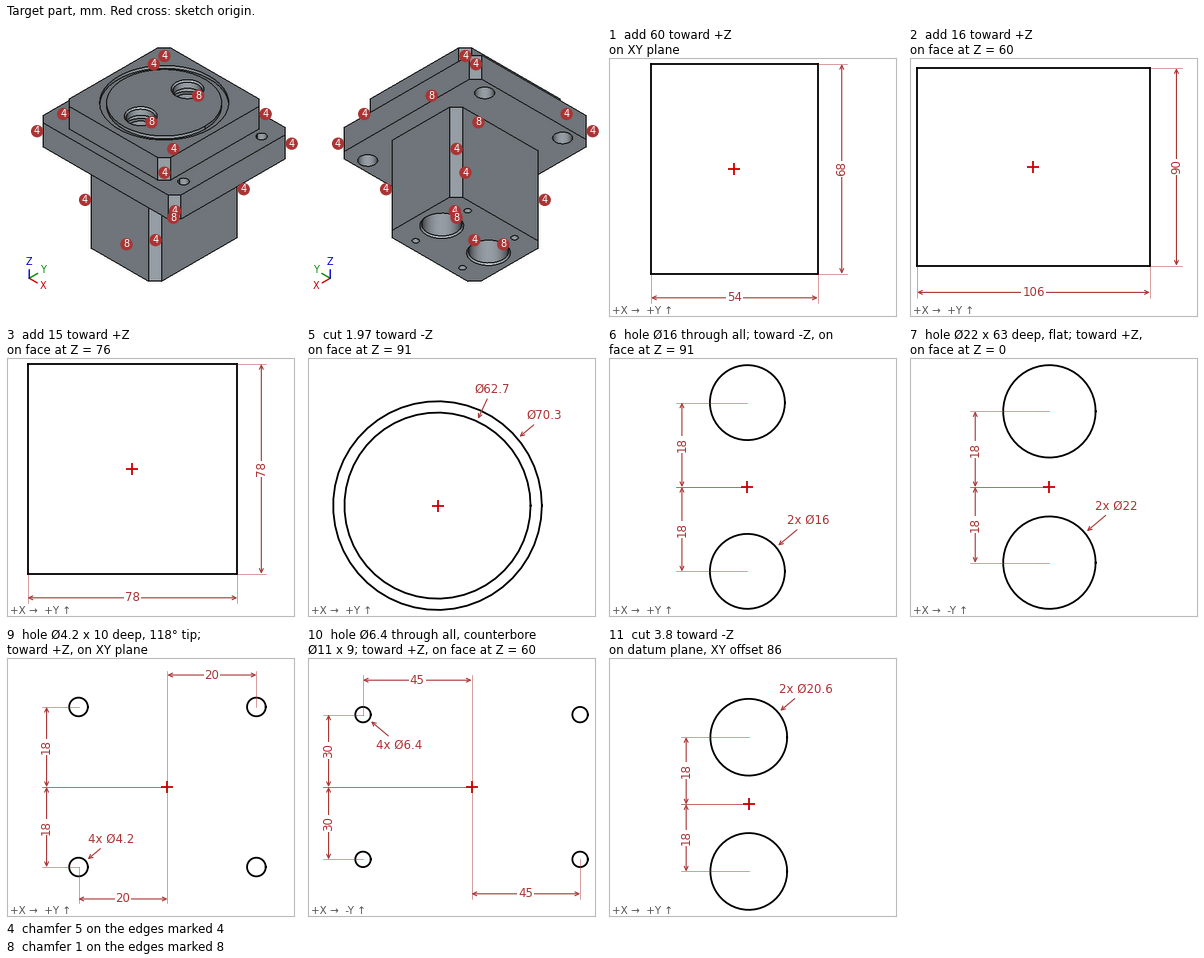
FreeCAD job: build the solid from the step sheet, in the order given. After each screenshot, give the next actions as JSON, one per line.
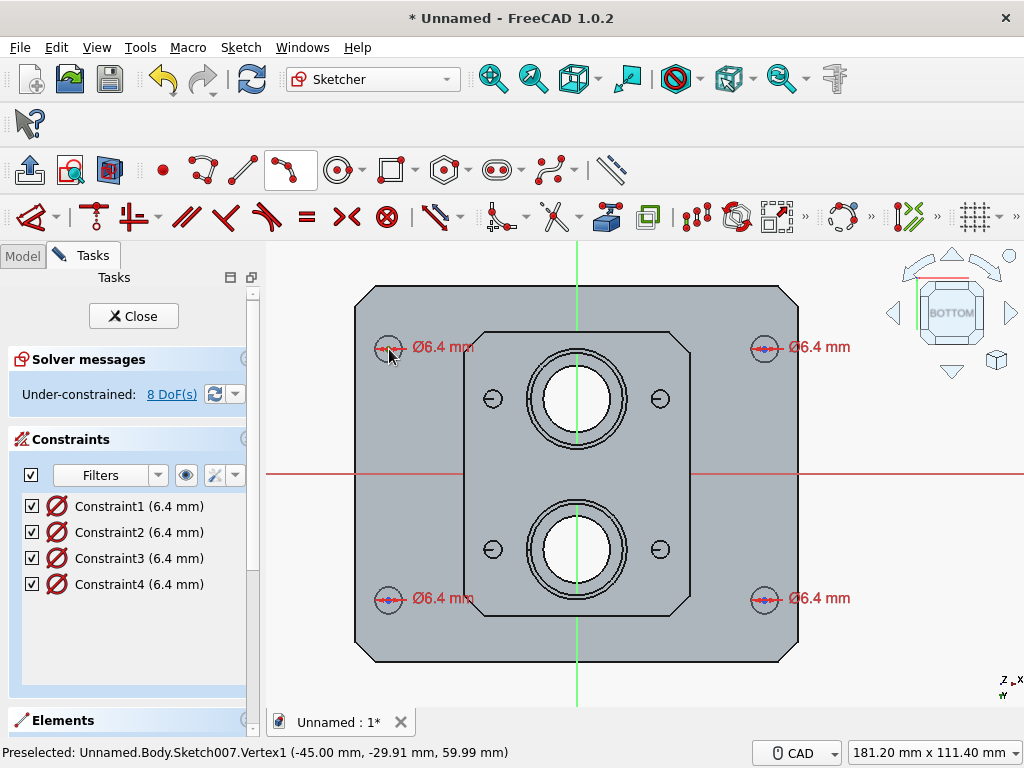
{"action": "left_click", "coordinate": [389, 600]}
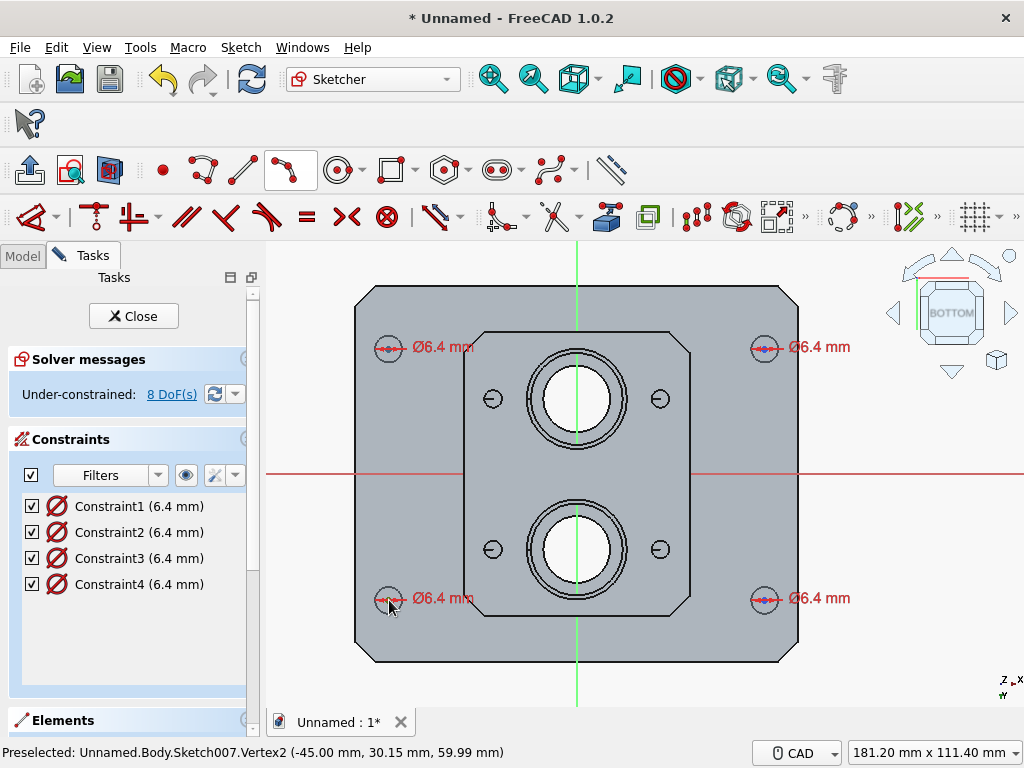
{"action": "key", "text": "v"}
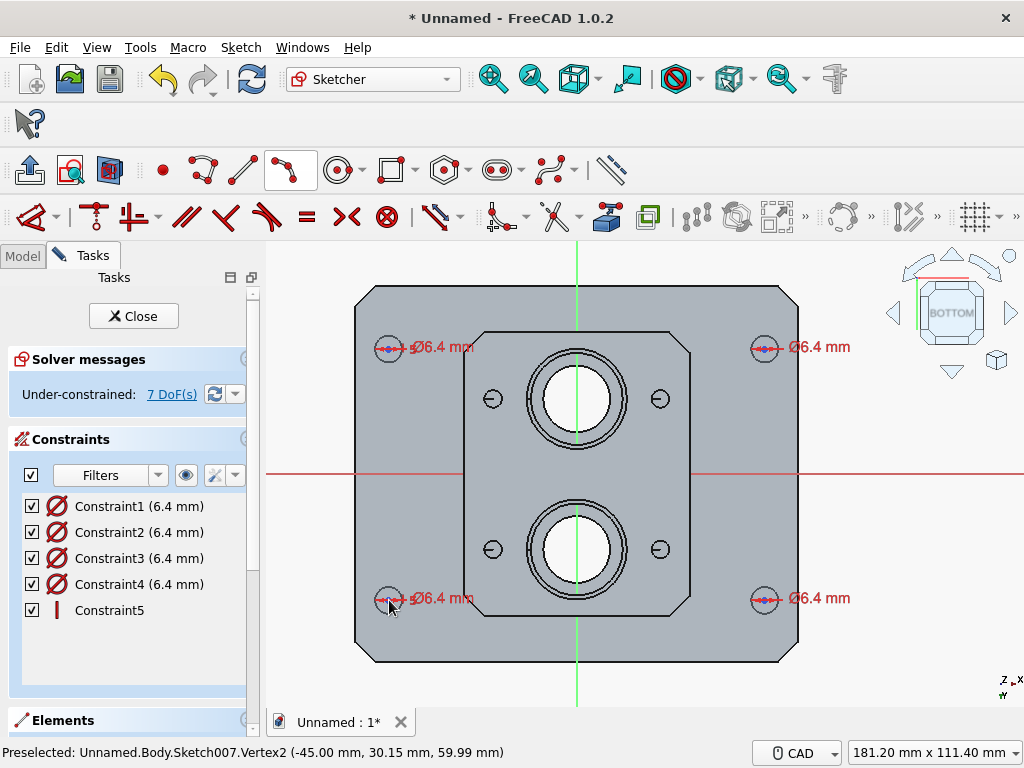
{"action": "left_click", "coordinate": [389, 600]}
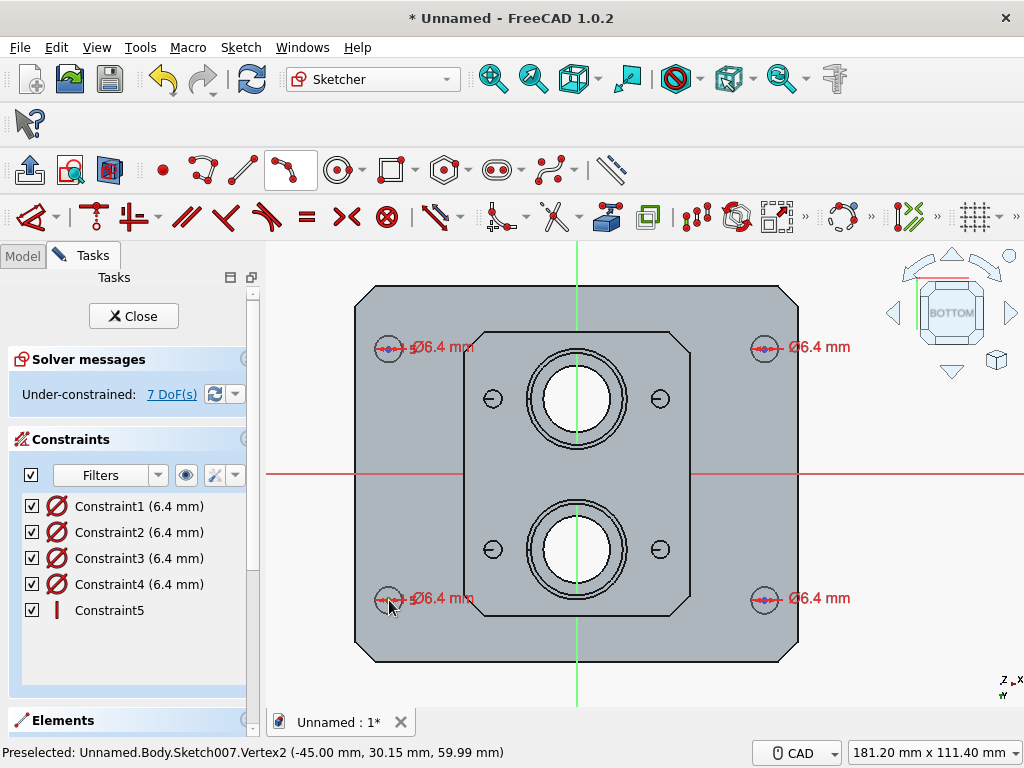
{"action": "left_click", "coordinate": [765, 600]}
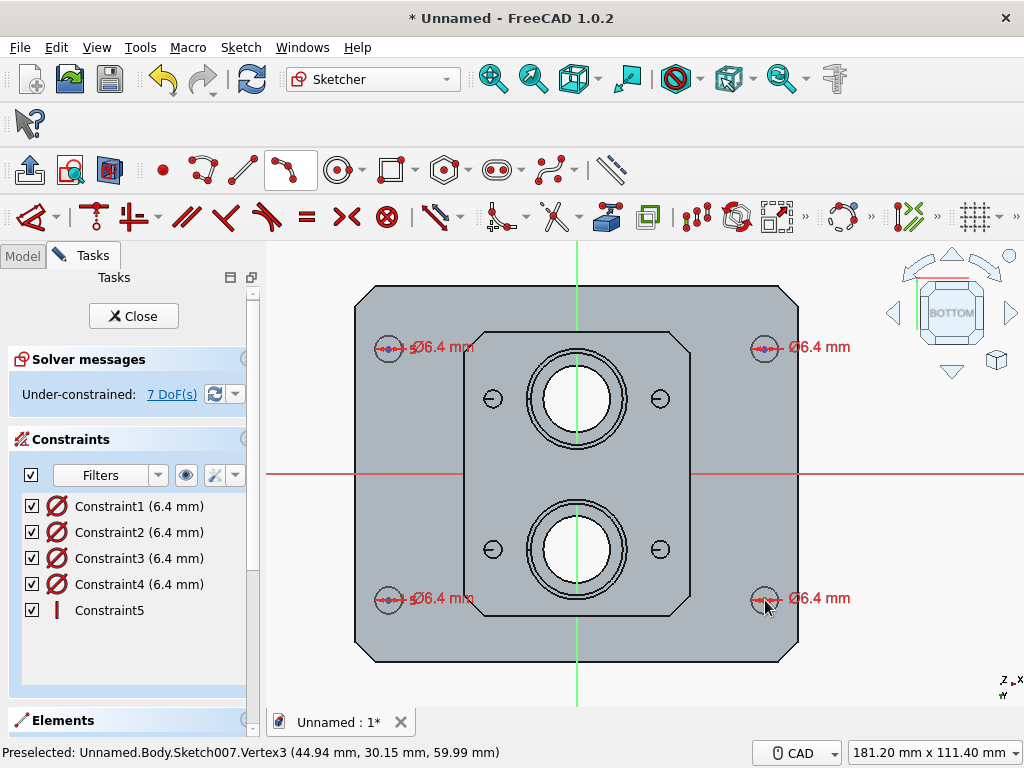
{"action": "key", "text": "h"}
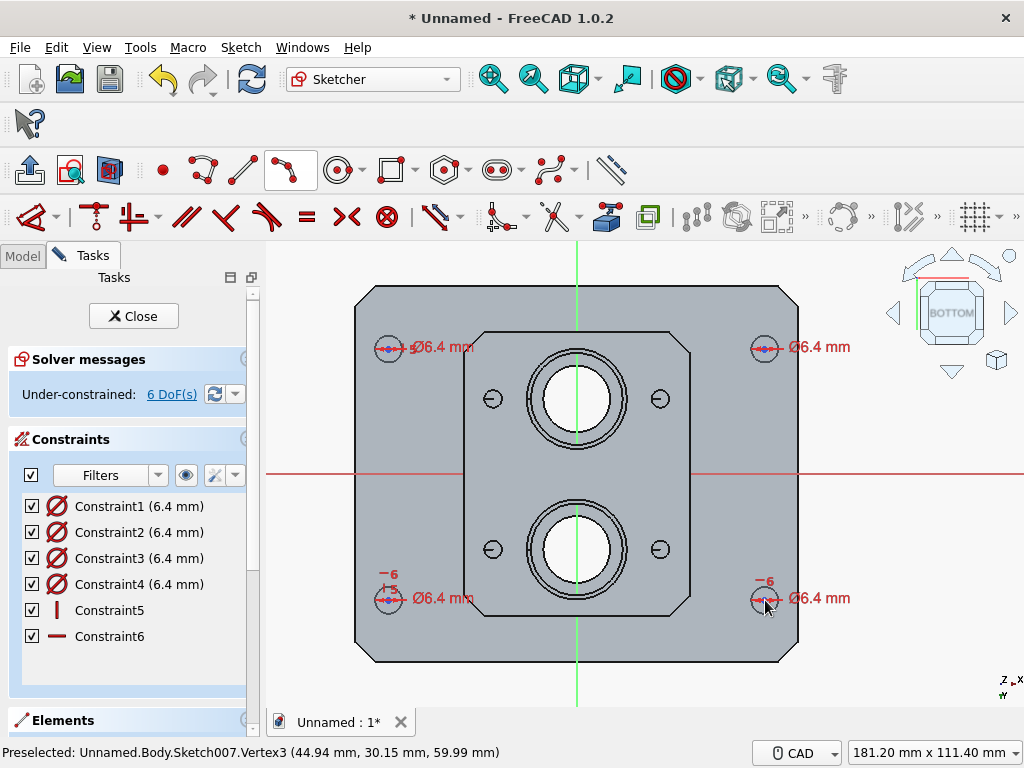
{"action": "left_click", "coordinate": [765, 600]}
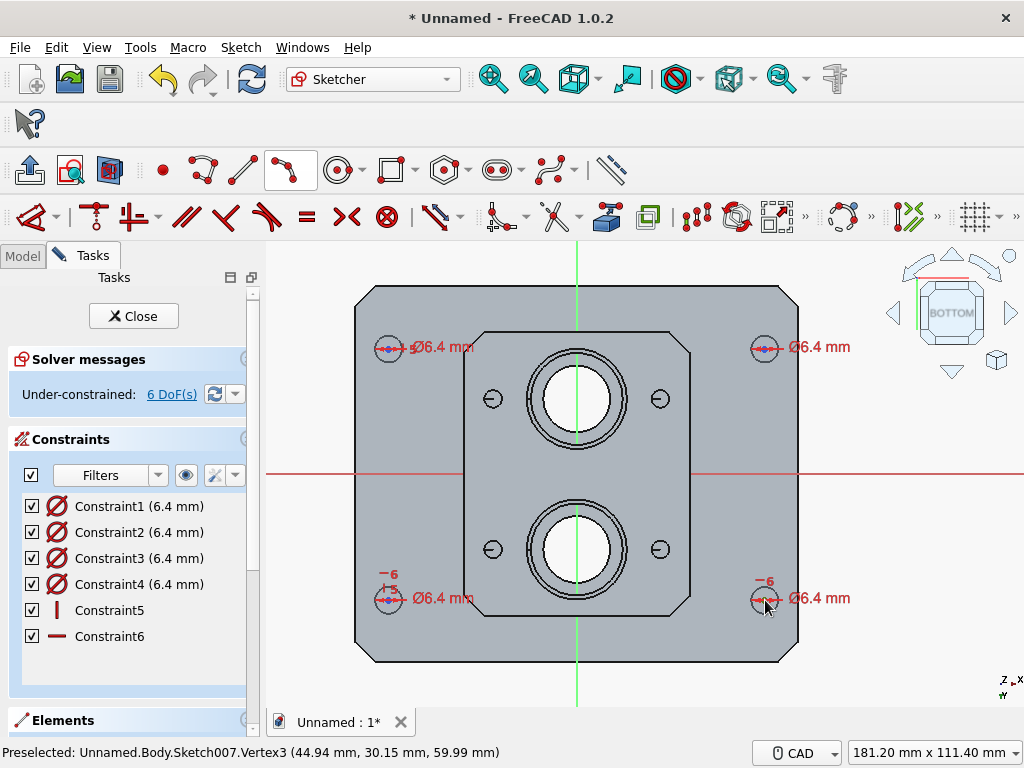
{"action": "left_click", "coordinate": [765, 349]}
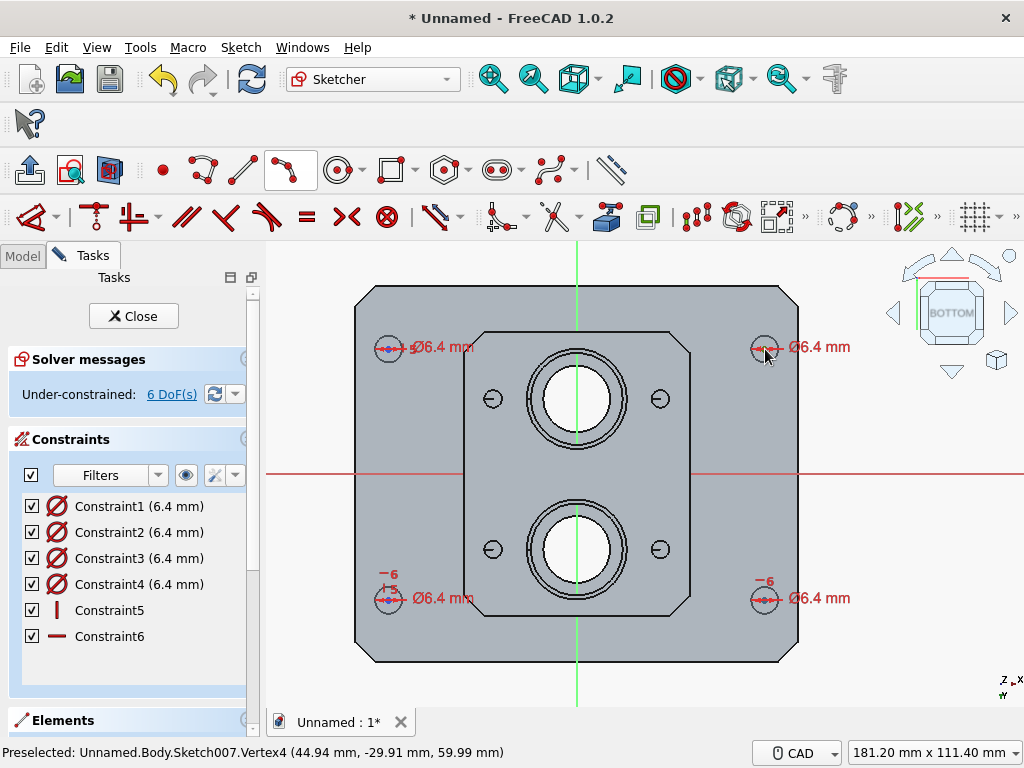
{"action": "key", "text": "v"}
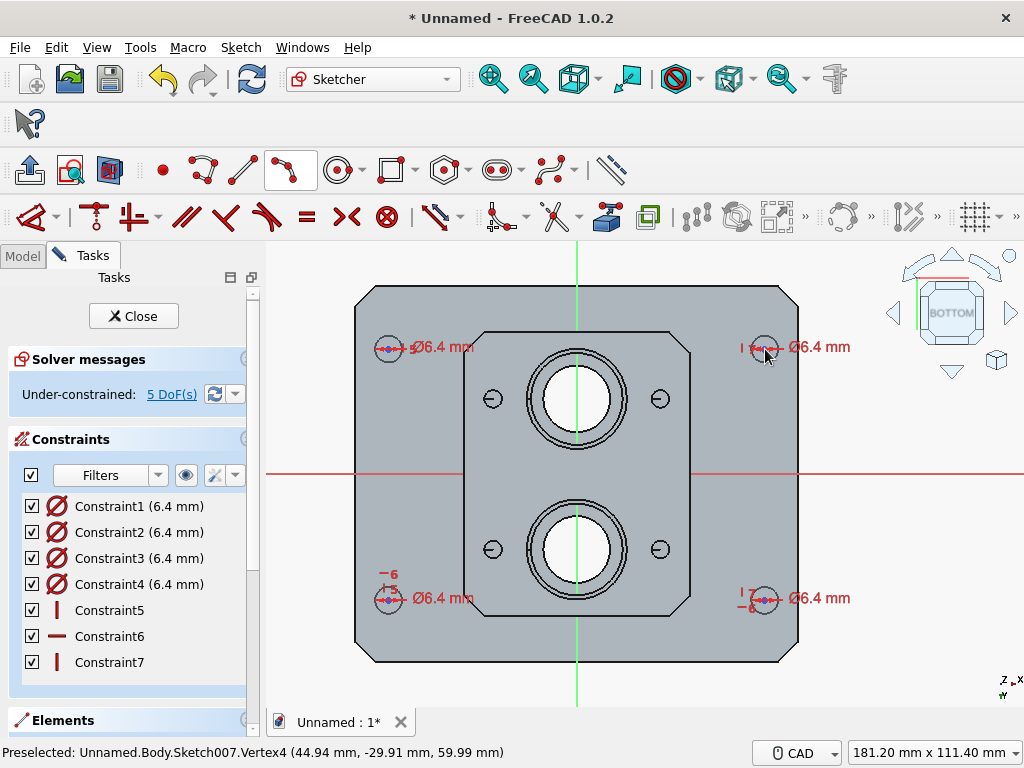
{"action": "left_click", "coordinate": [389, 349]}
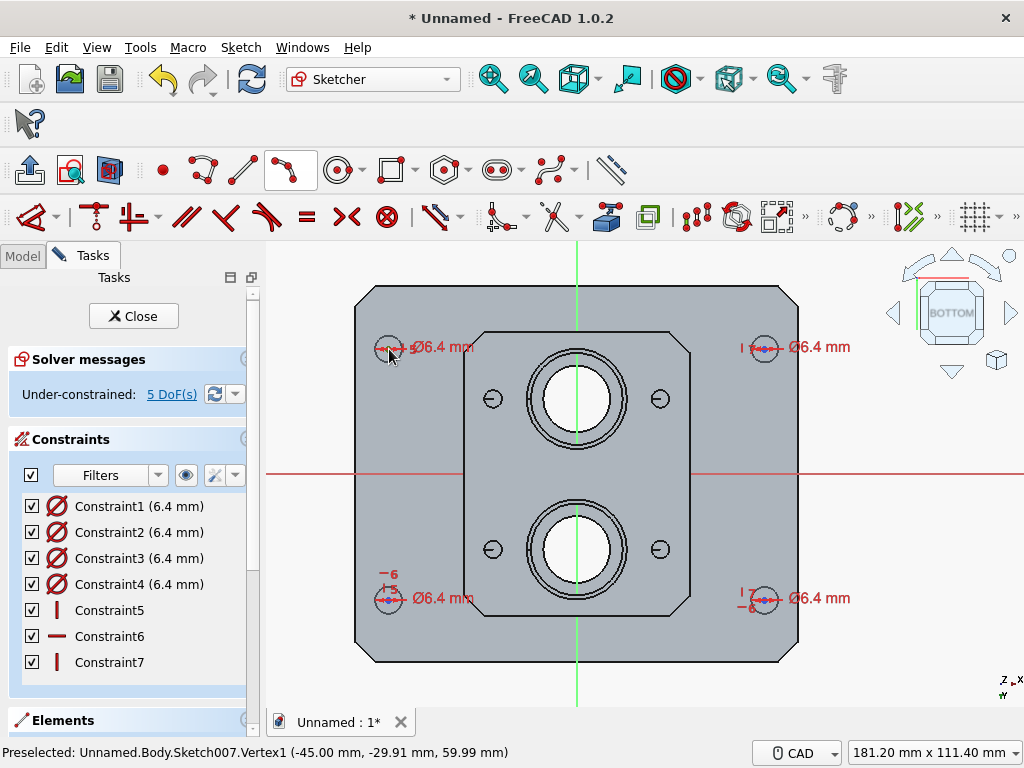
{"action": "left_click", "coordinate": [765, 349]}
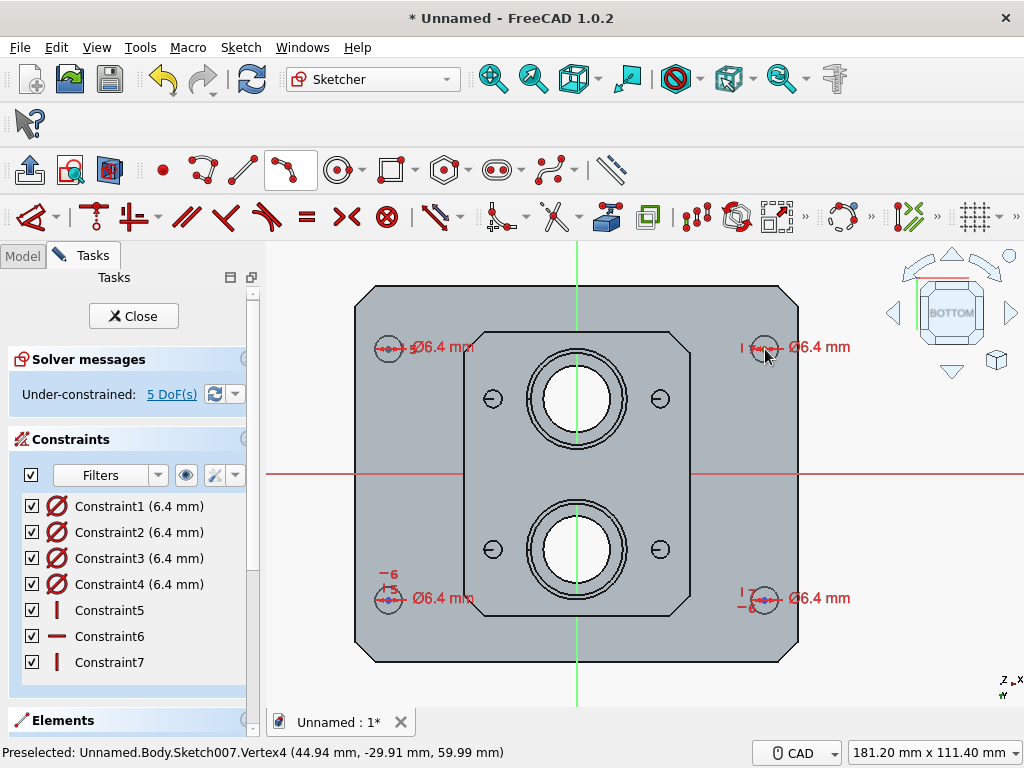
{"action": "key", "text": "h"}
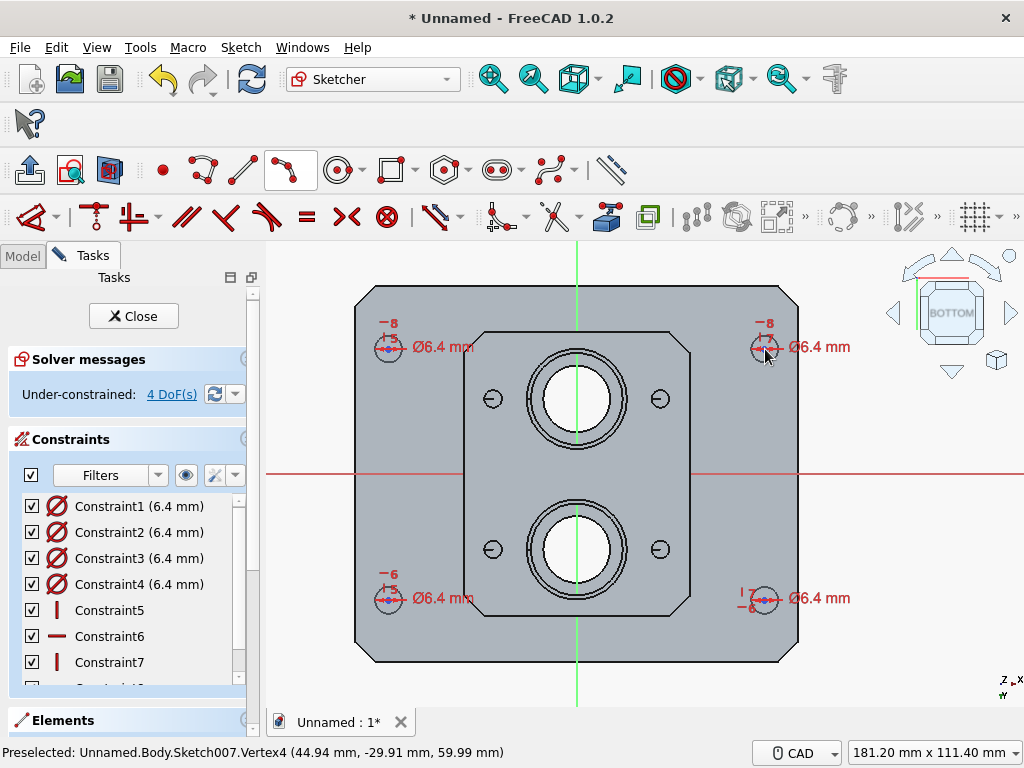
{"action": "left_click", "coordinate": [32, 218]}